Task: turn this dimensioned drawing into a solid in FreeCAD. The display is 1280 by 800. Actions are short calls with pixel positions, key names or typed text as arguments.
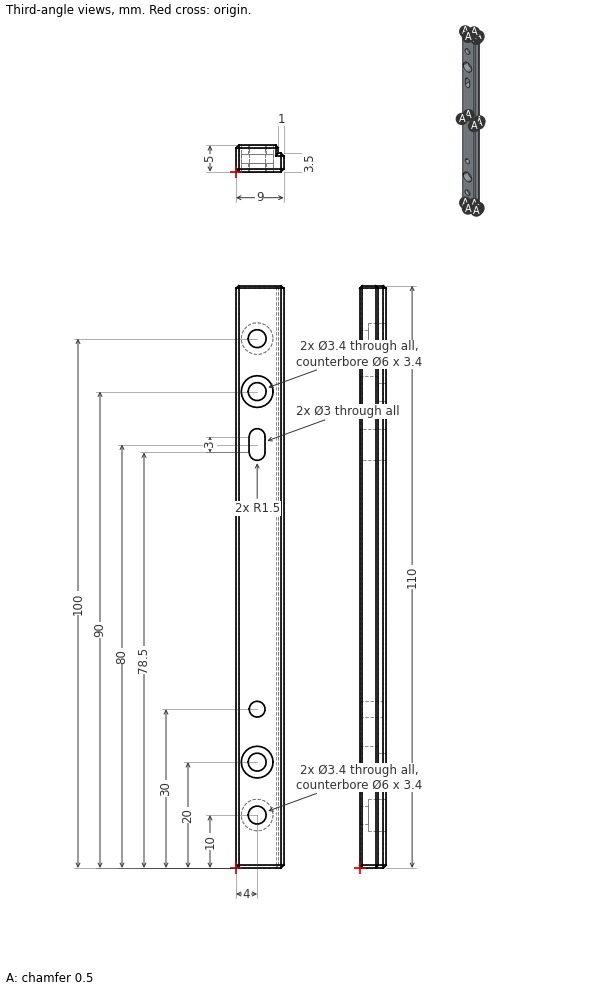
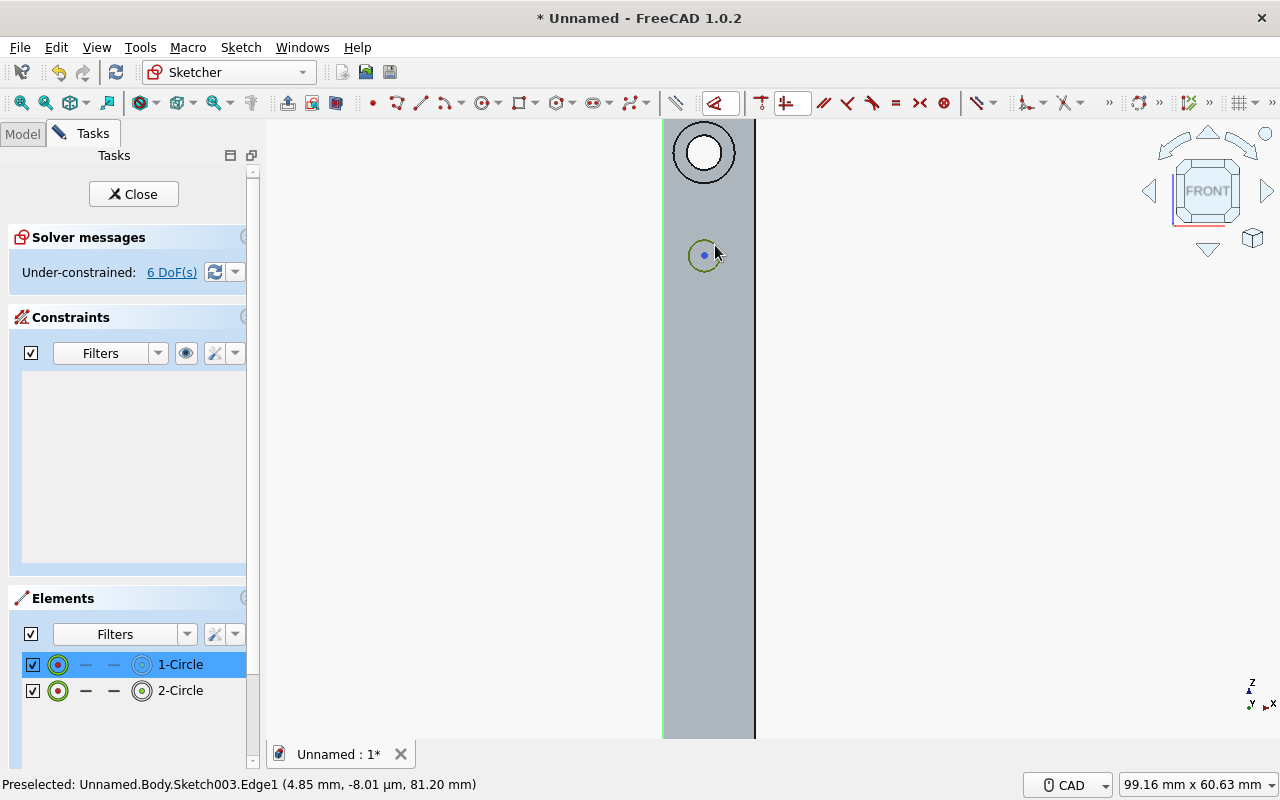
scroll(715, 244, down, 4)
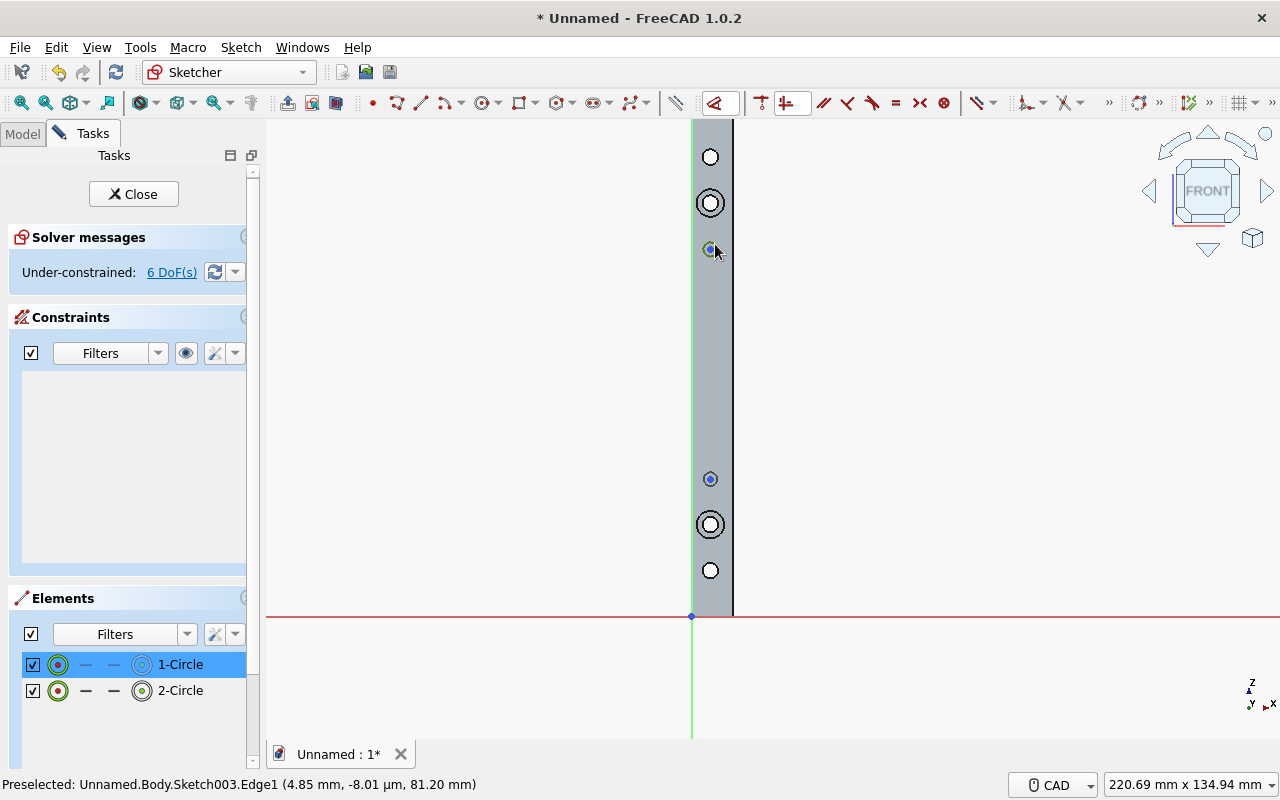
scroll(715, 474, up, 4)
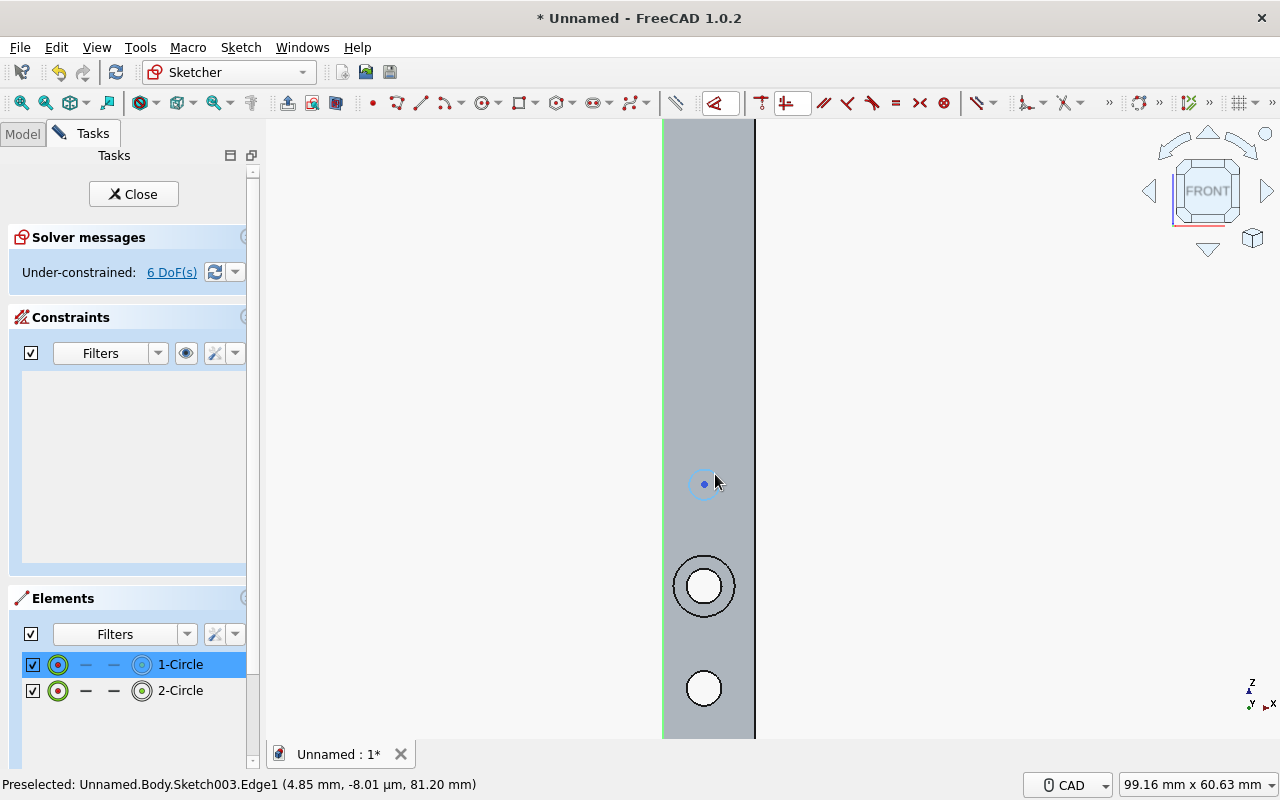
click(715, 474)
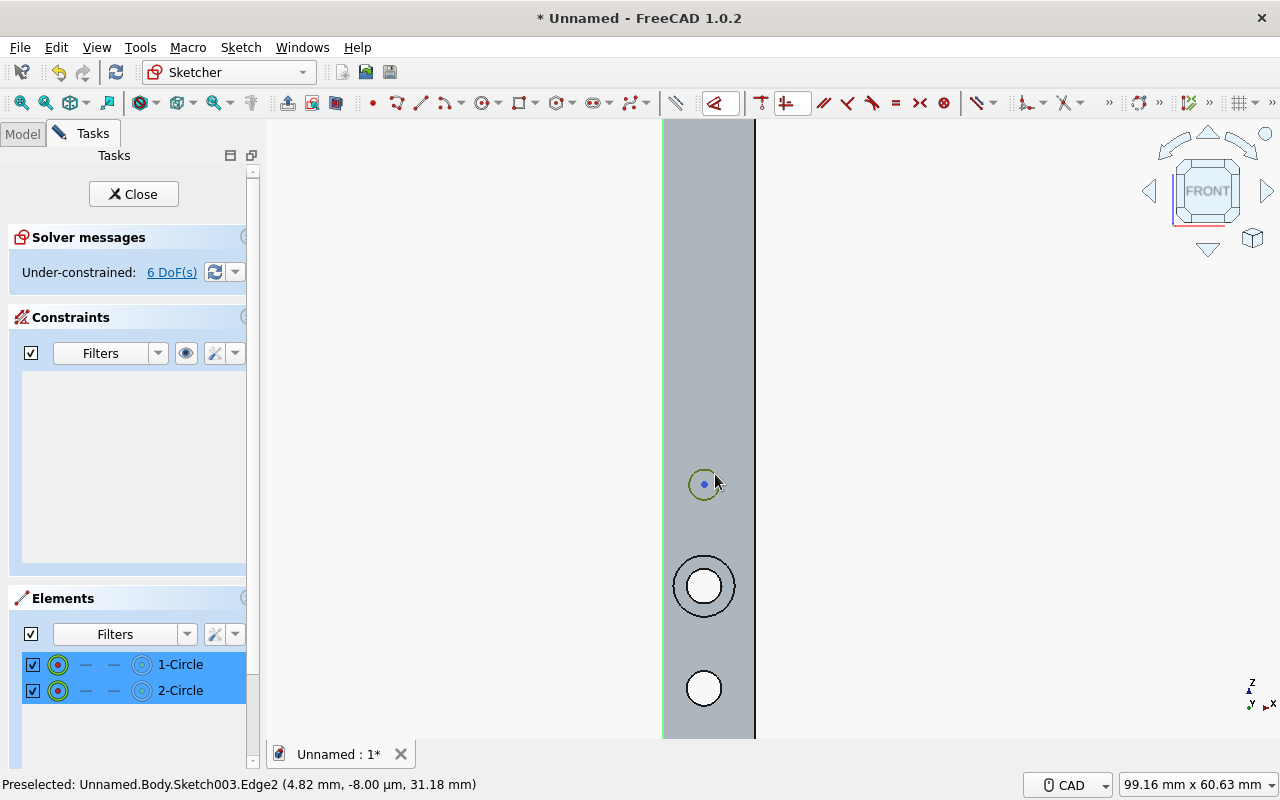
click(896, 104)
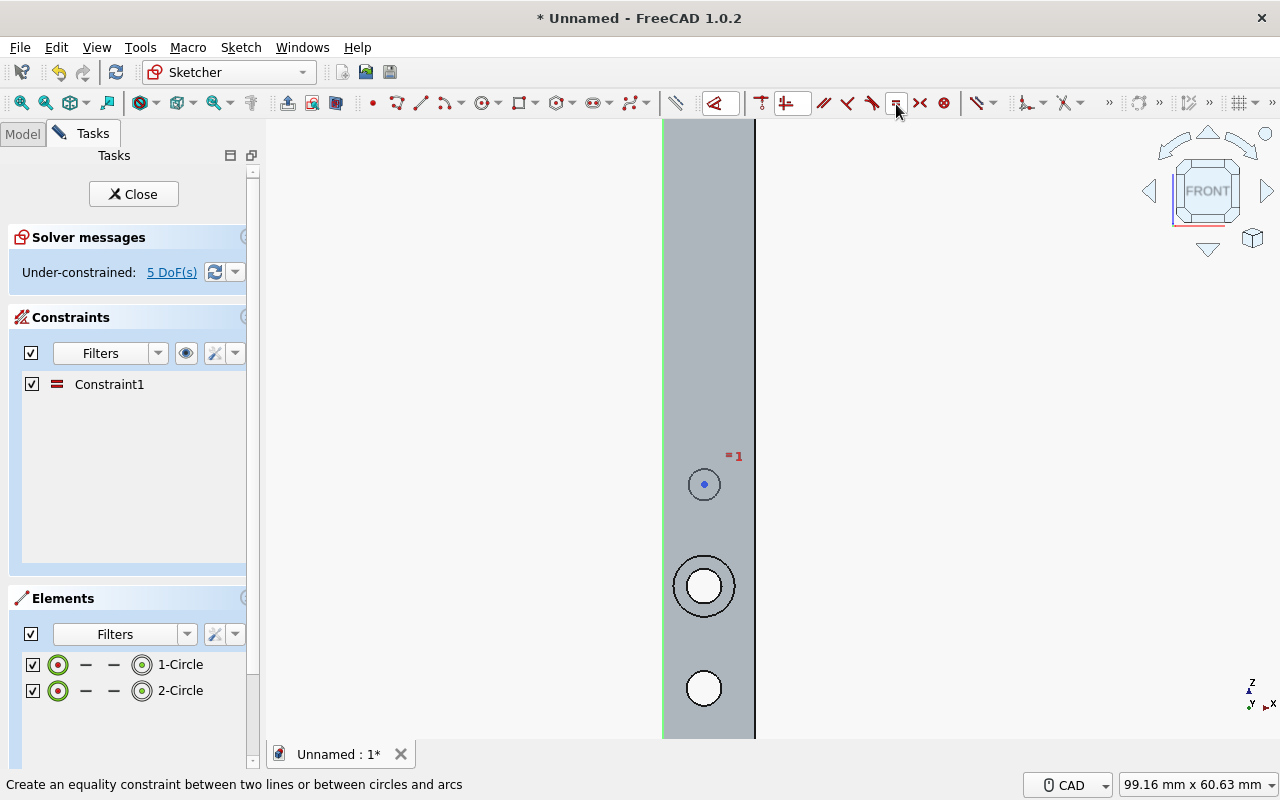
key(d)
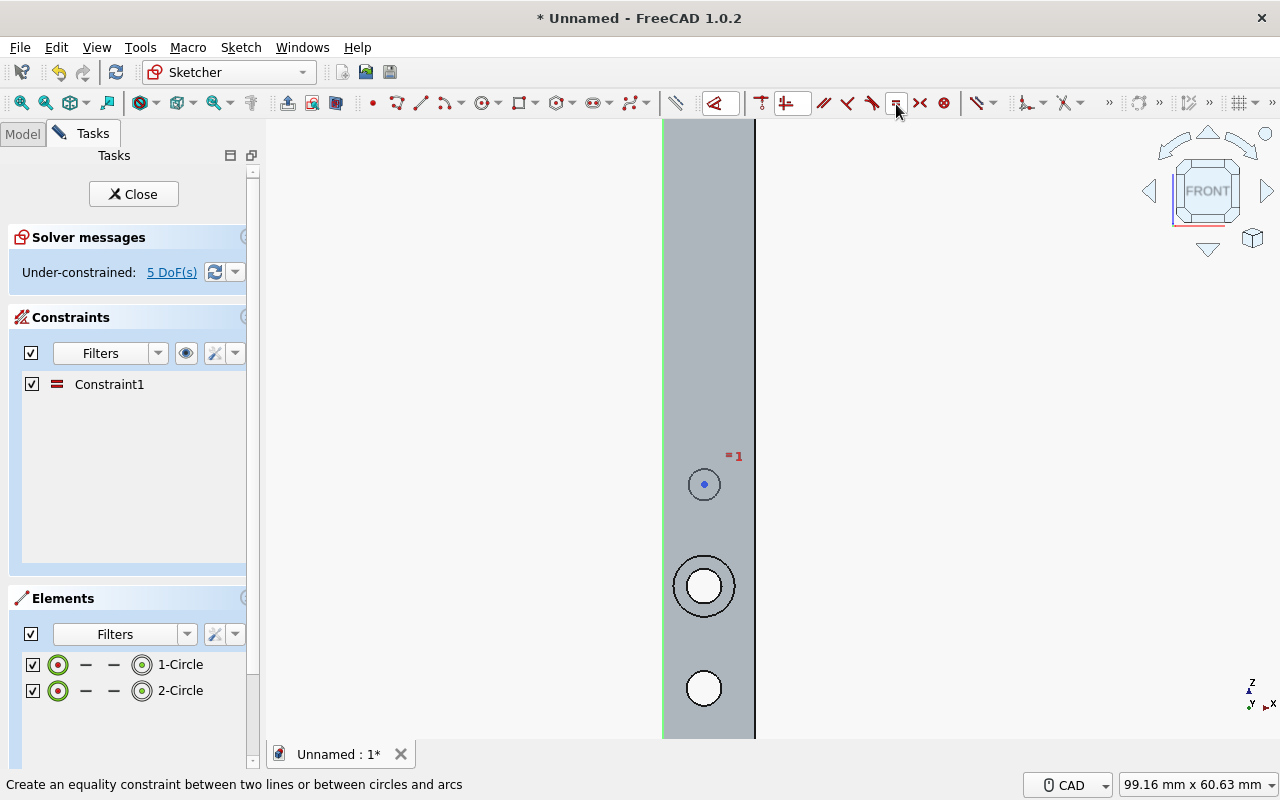
scroll(715, 474, down, 4)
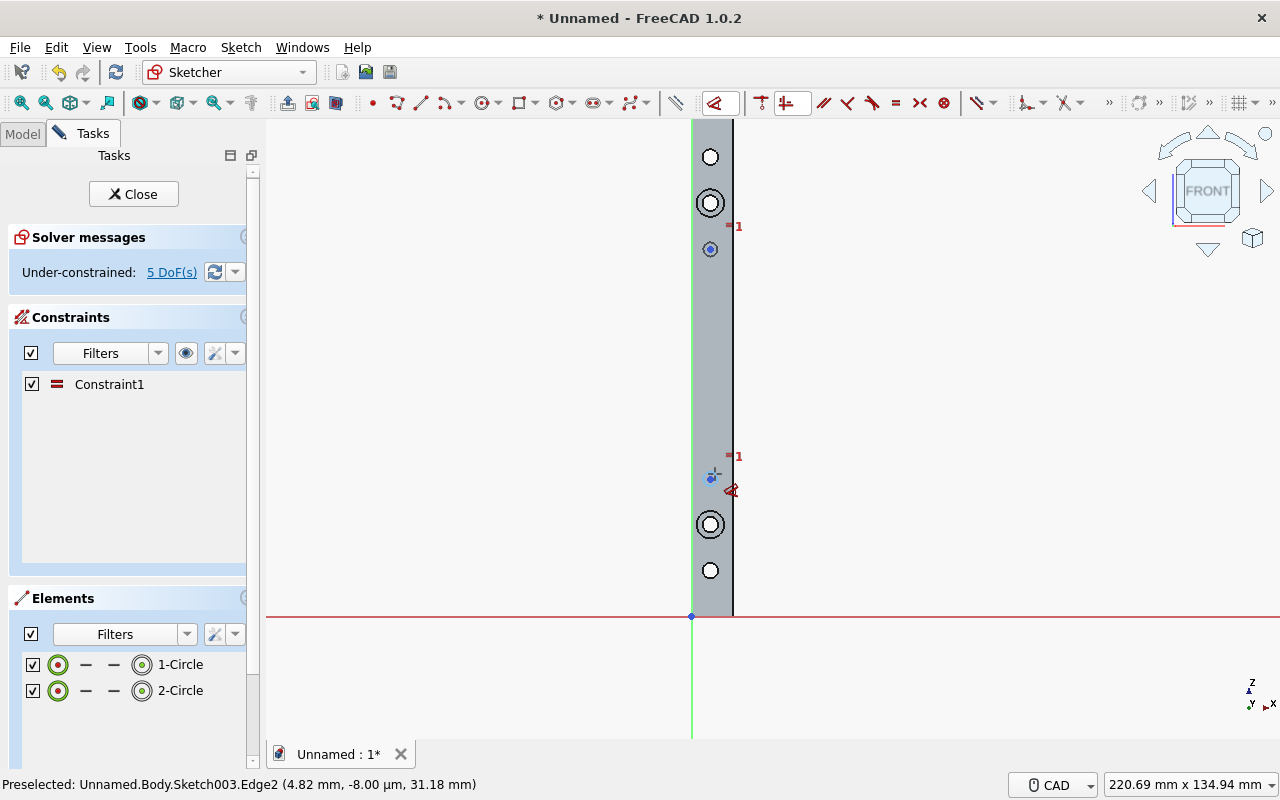
scroll(715, 244, up, 6)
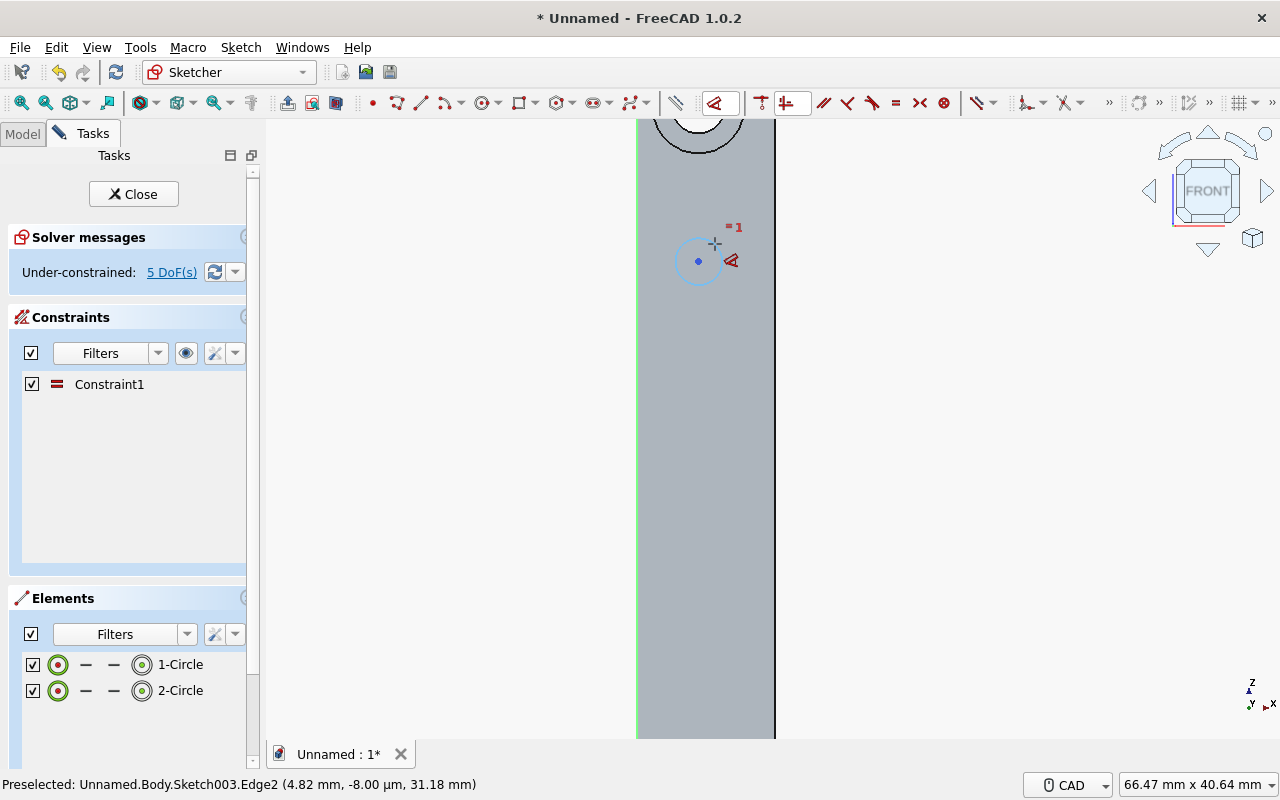
click(715, 245)
click(737, 222)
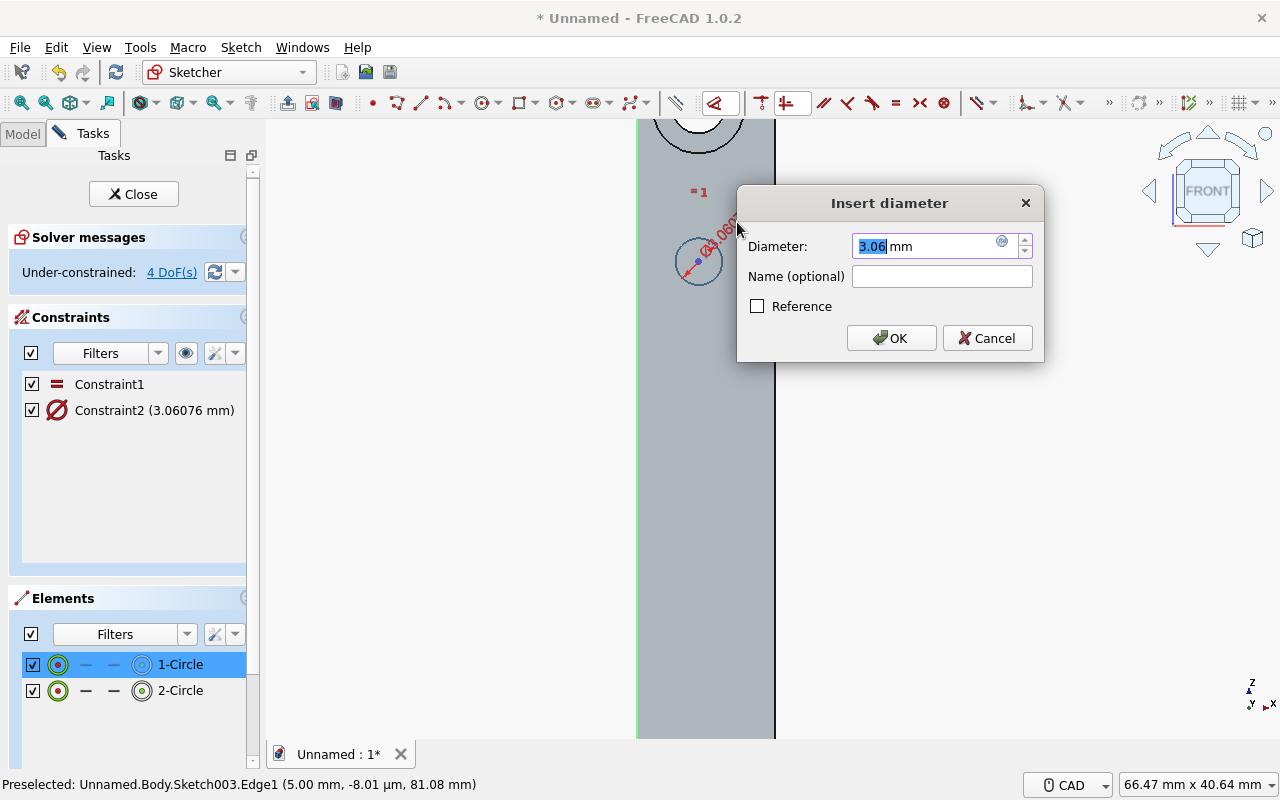
text(3)
key(Return)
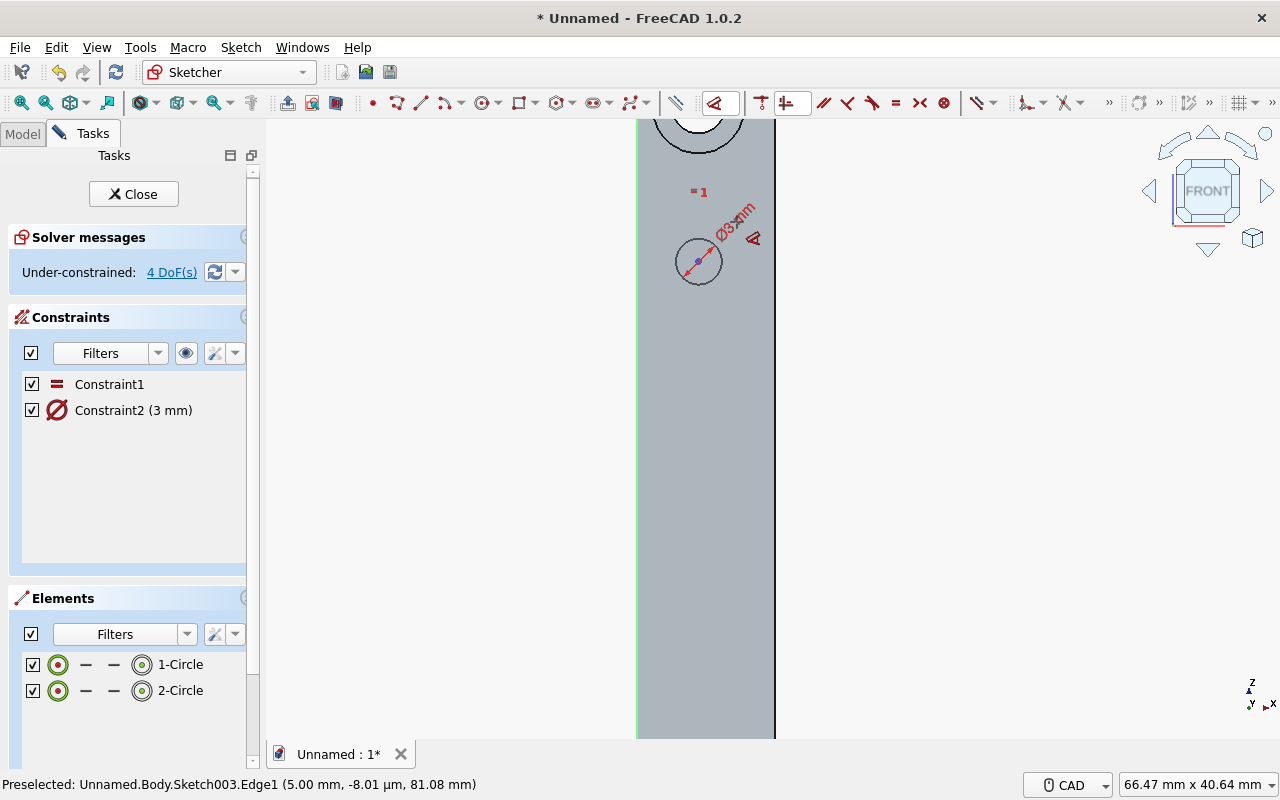
click(699, 262)
click(654, 228)